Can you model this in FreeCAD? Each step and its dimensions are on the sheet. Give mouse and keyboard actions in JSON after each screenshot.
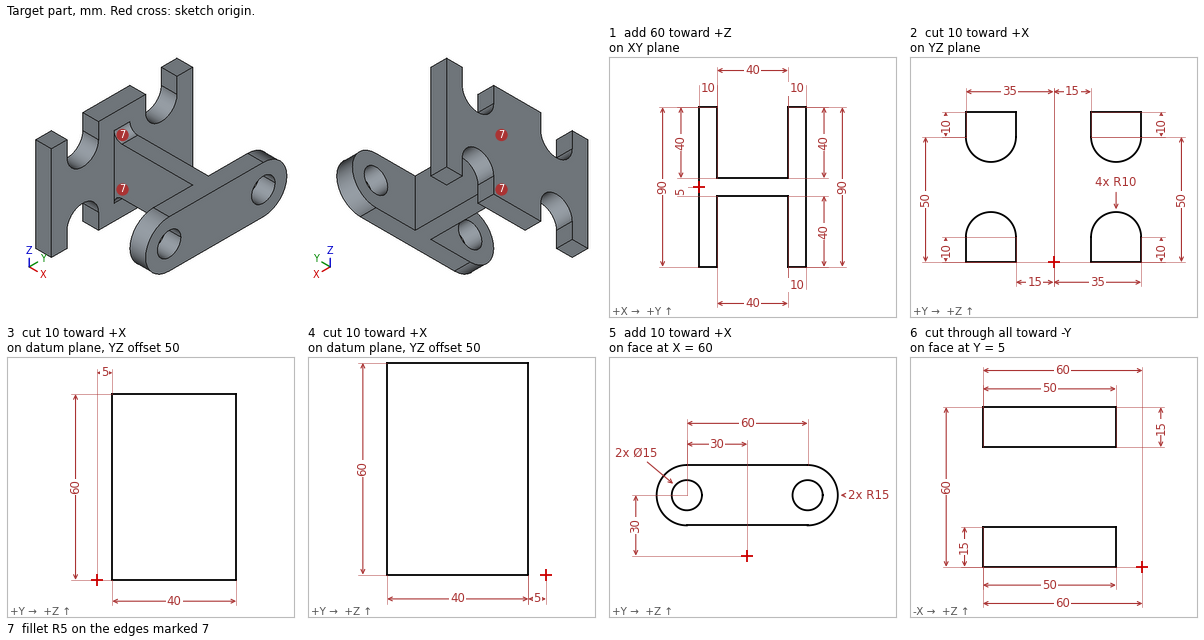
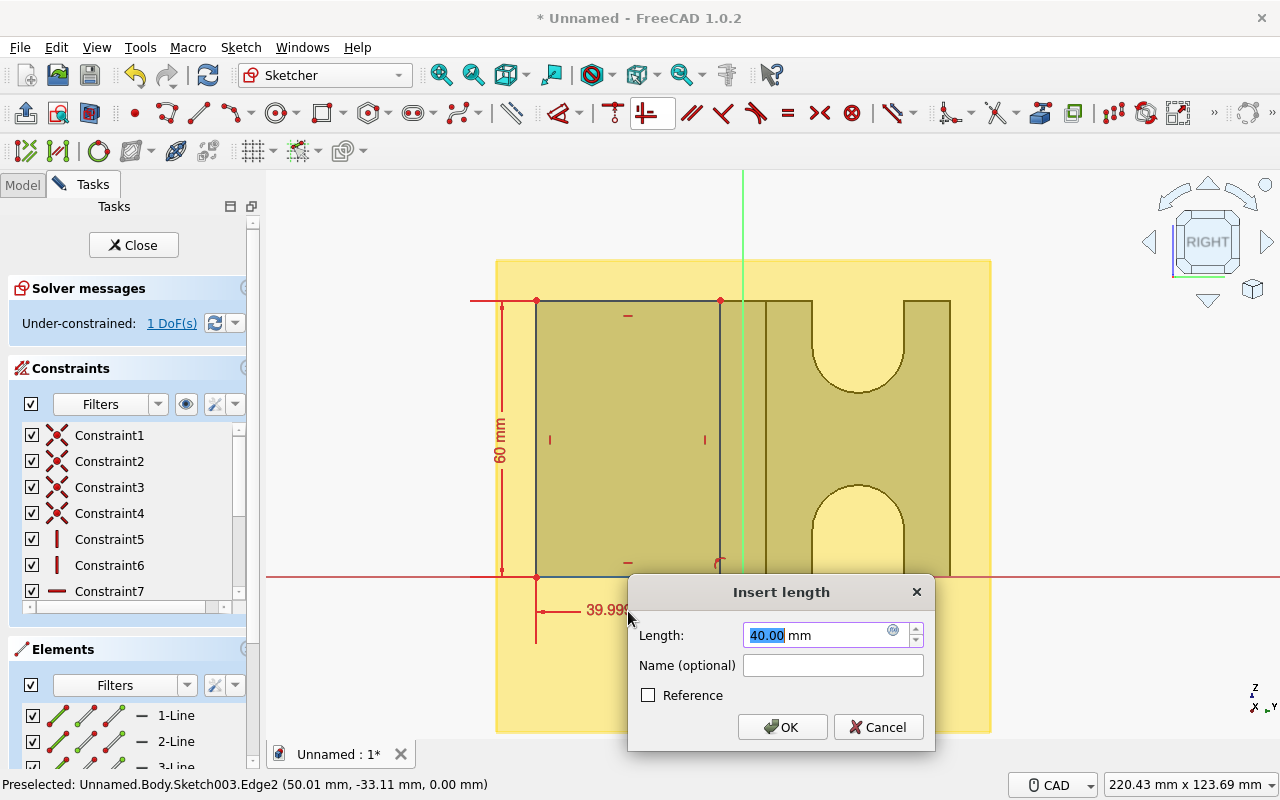
{"action": "type", "text": "40"}
{"action": "key", "text": "Return"}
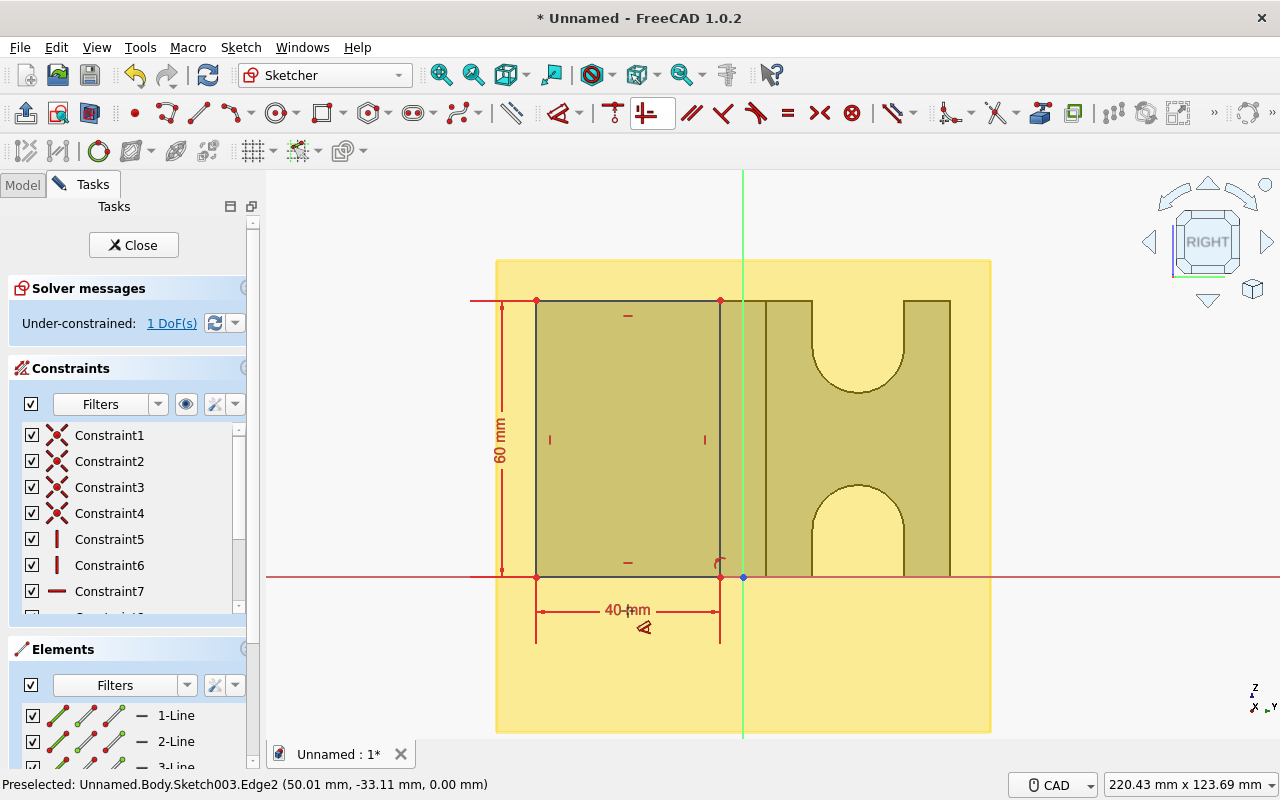
{"action": "scroll", "coordinate": [720, 577], "scroll_direction": "up", "scroll_amount": 3}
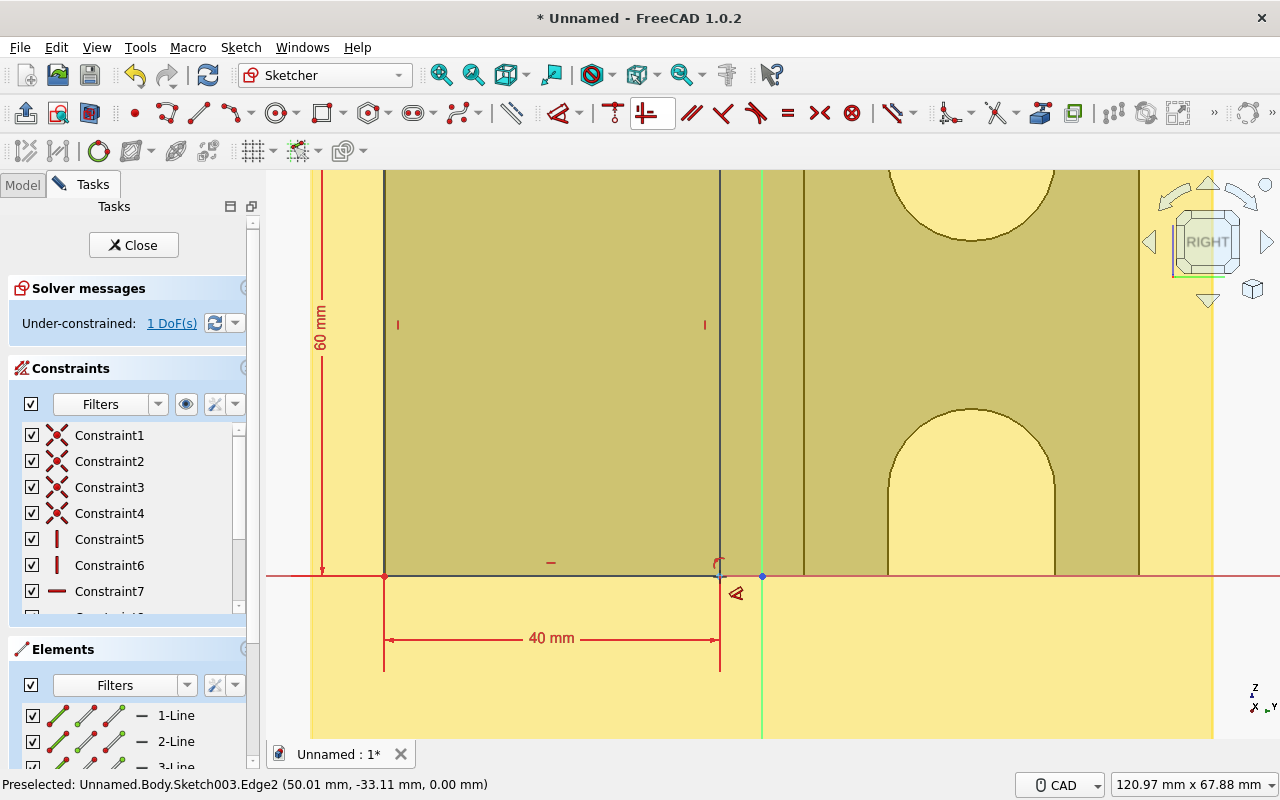
{"action": "left_click", "coordinate": [720, 576]}
{"action": "left_click", "coordinate": [741, 610]}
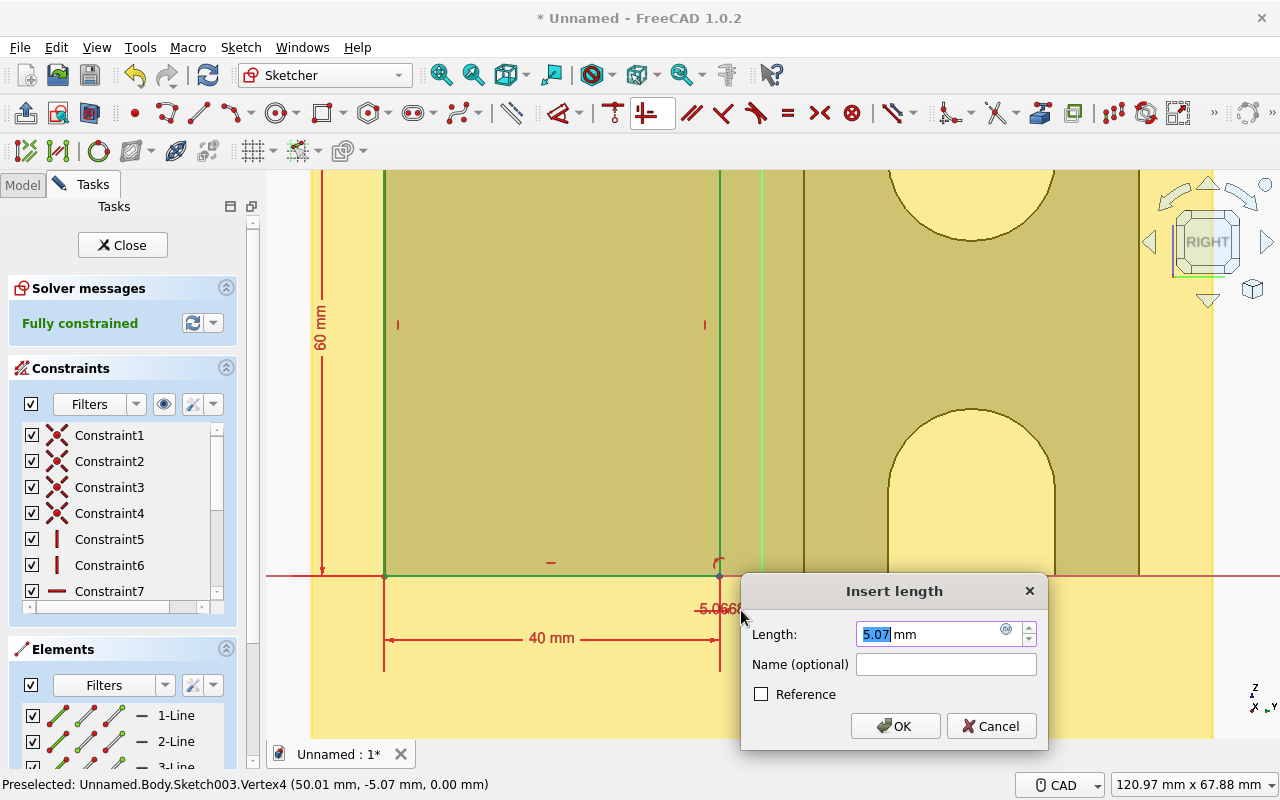
{"action": "type", "text": "5"}
{"action": "key", "text": "Return"}
{"action": "key", "text": "Escape"}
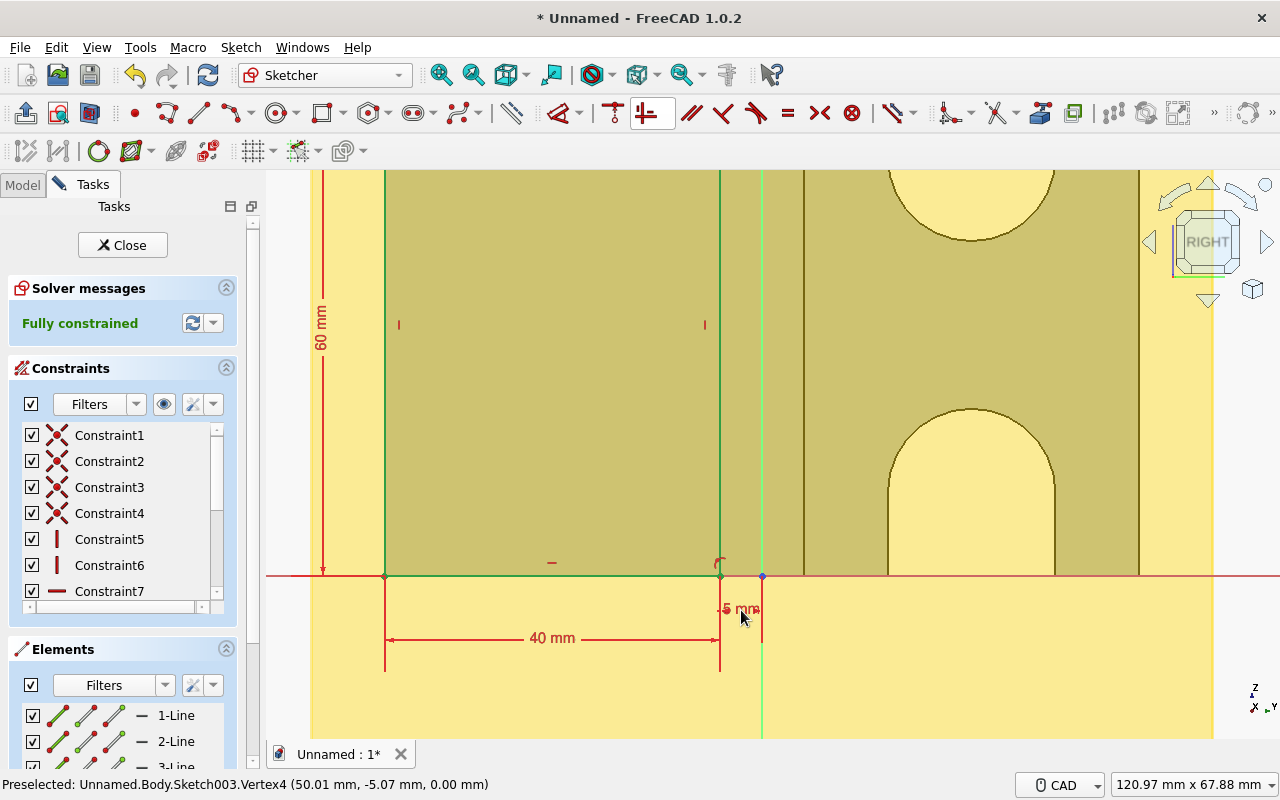
{"action": "left_click", "coordinate": [123, 245]}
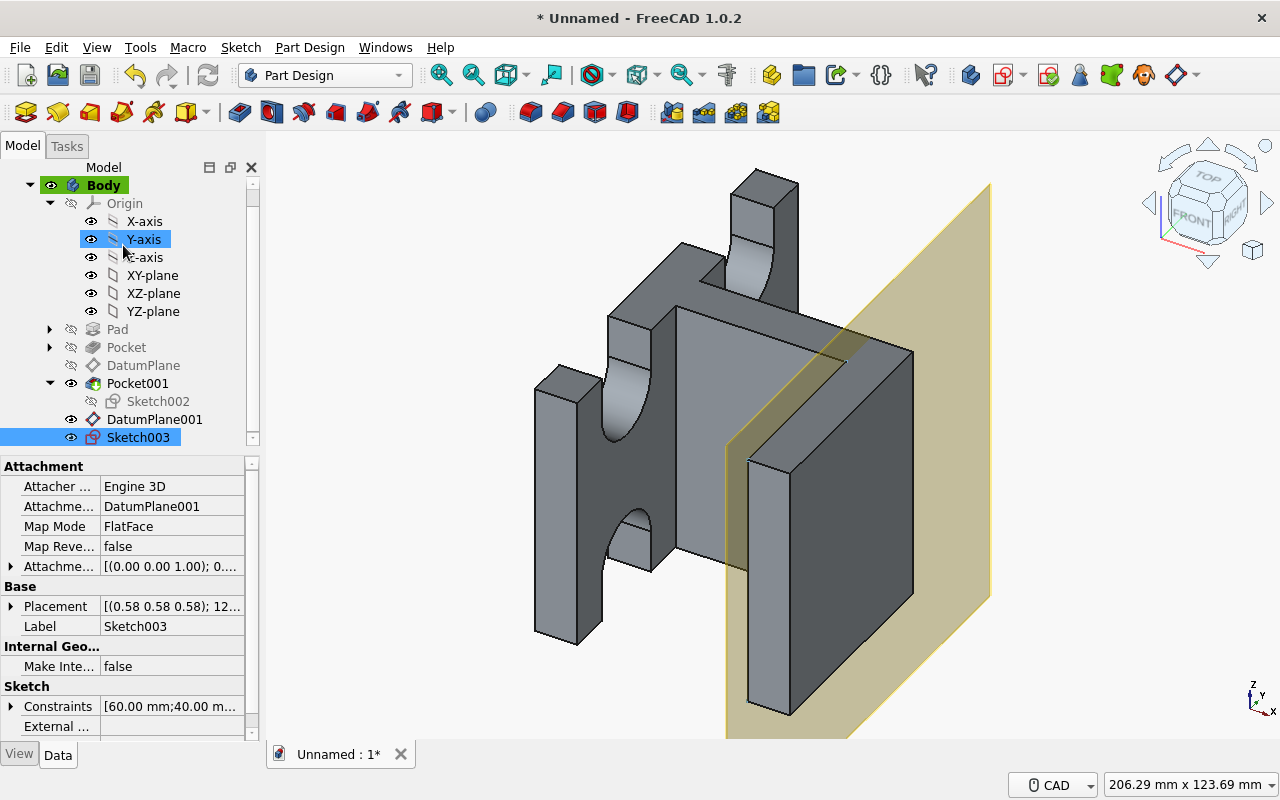
{"action": "left_click", "coordinate": [240, 112]}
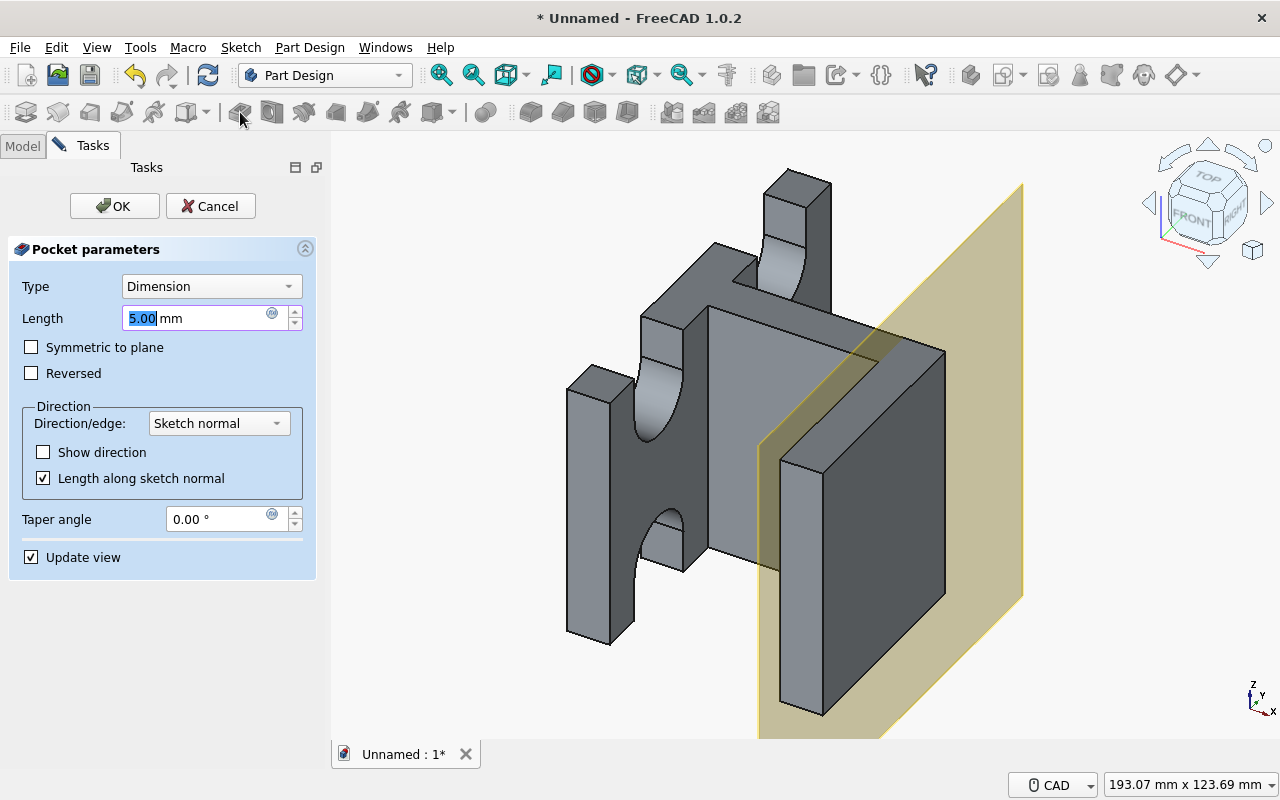
{"action": "type", "text": "10"}
{"action": "key", "text": "Tab"}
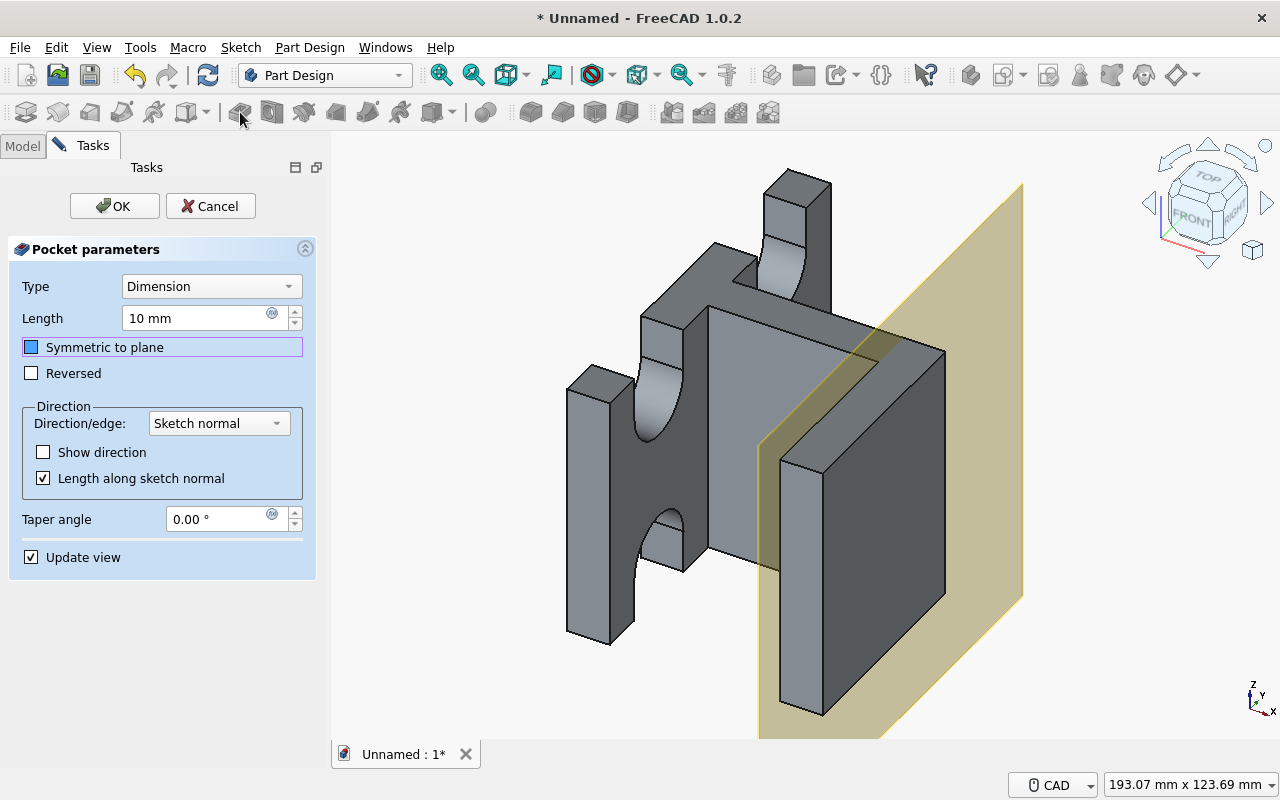
{"action": "left_click", "coordinate": [30, 373]}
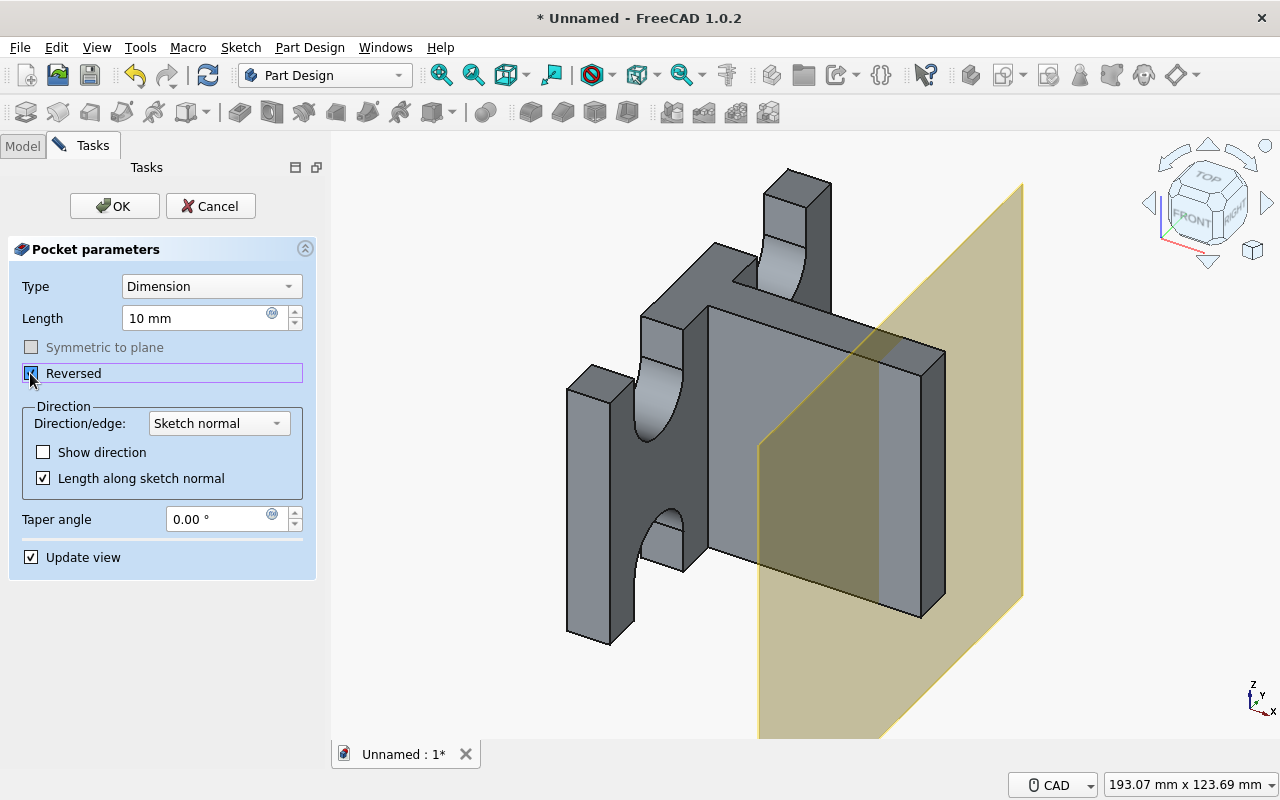
{"action": "left_click", "coordinate": [115, 206]}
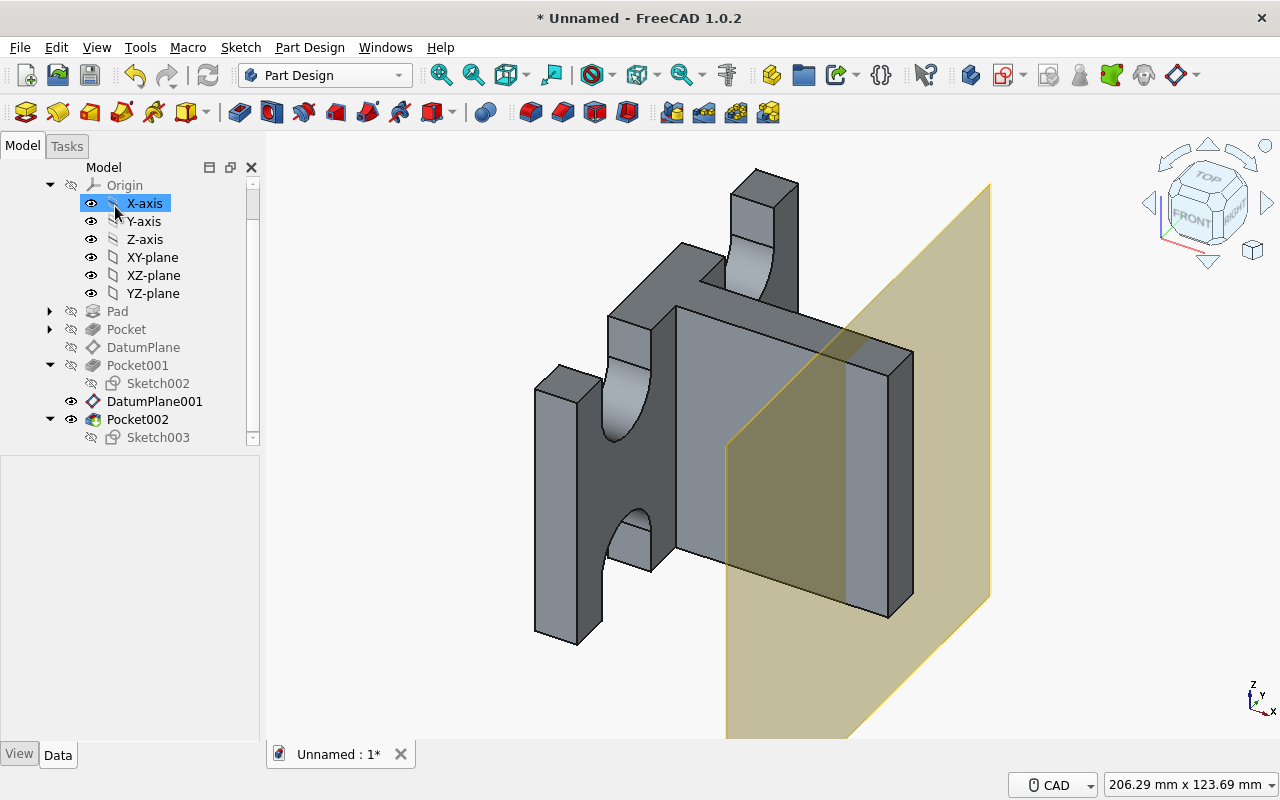
{"action": "left_click", "coordinate": [116, 401]}
{"action": "key", "text": "space"}